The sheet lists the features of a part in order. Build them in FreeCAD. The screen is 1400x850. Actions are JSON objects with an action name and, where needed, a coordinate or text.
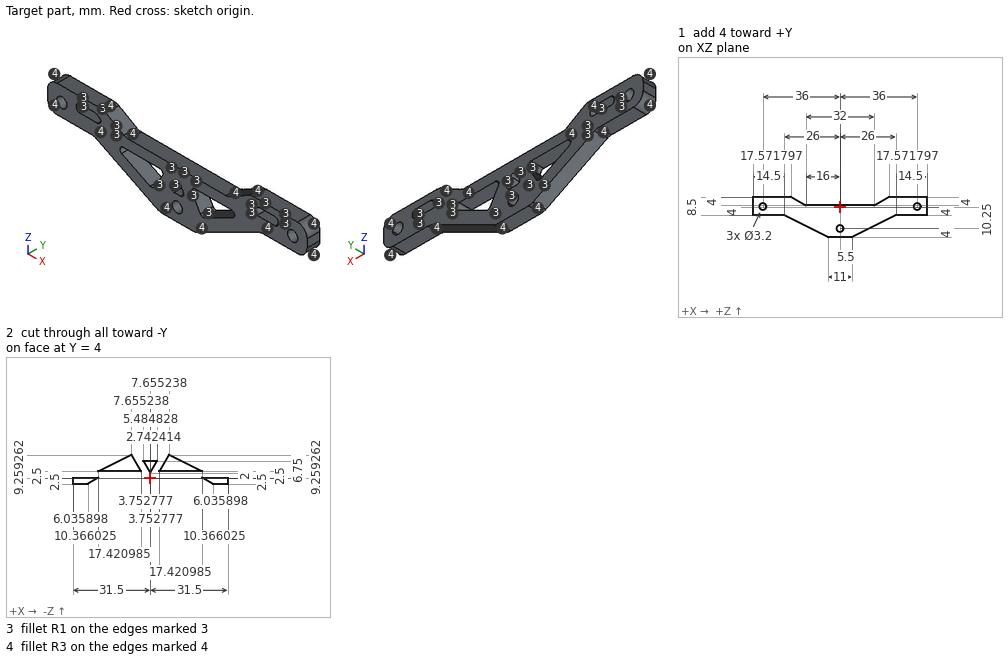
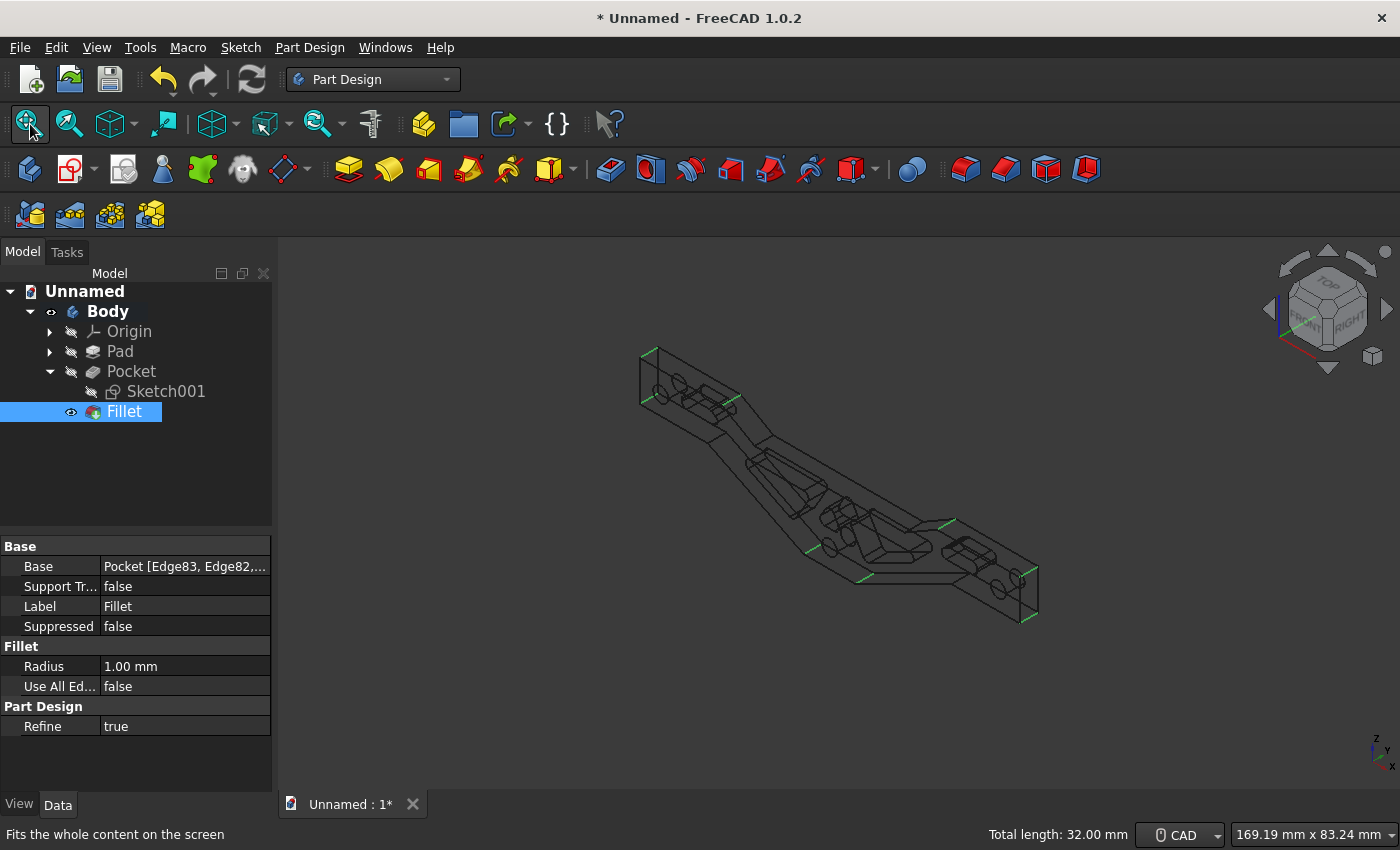
{"action": "left_click", "coordinate": [918, 524], "text": "ctrl"}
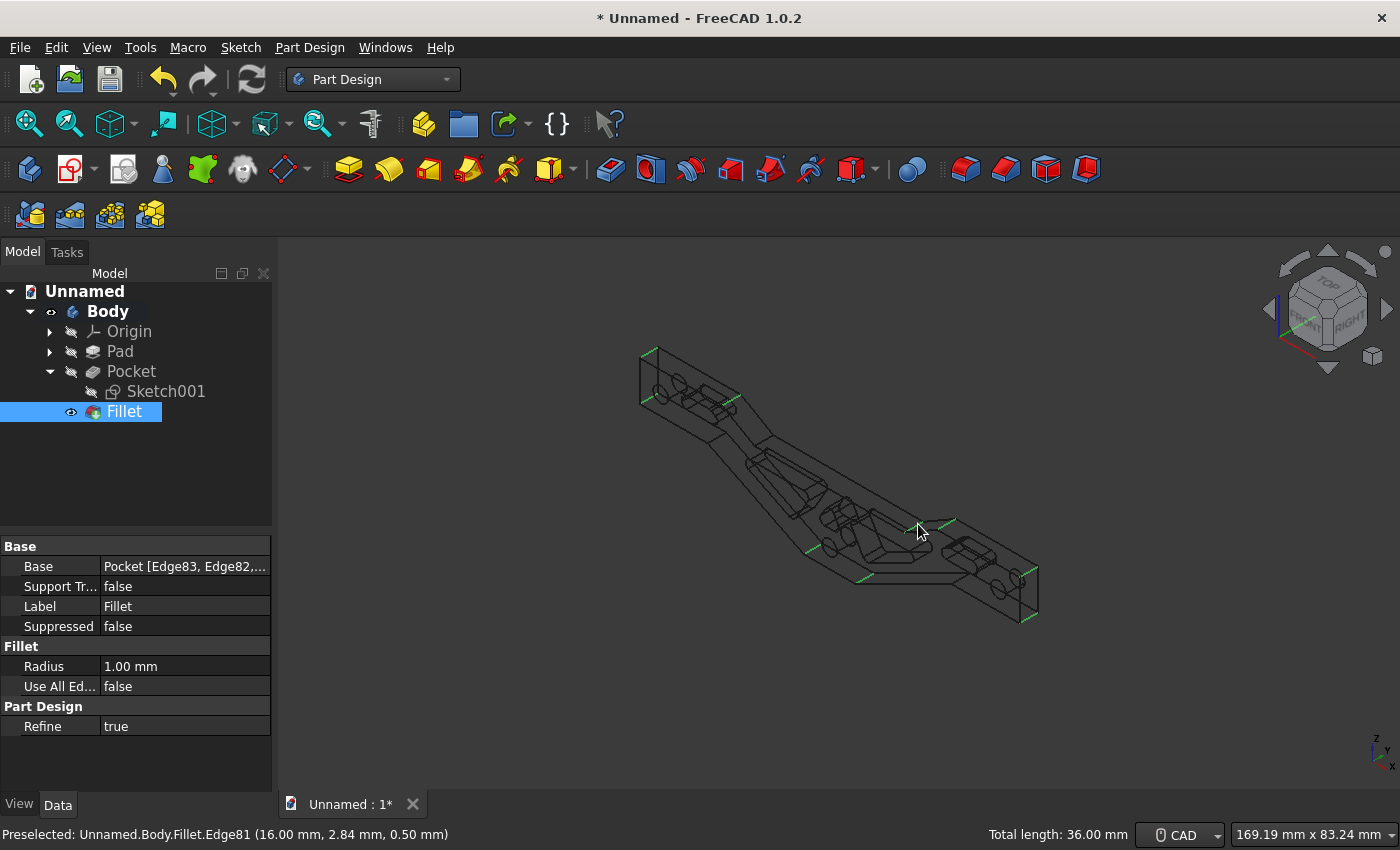
{"action": "left_click", "coordinate": [764, 440], "text": "ctrl"}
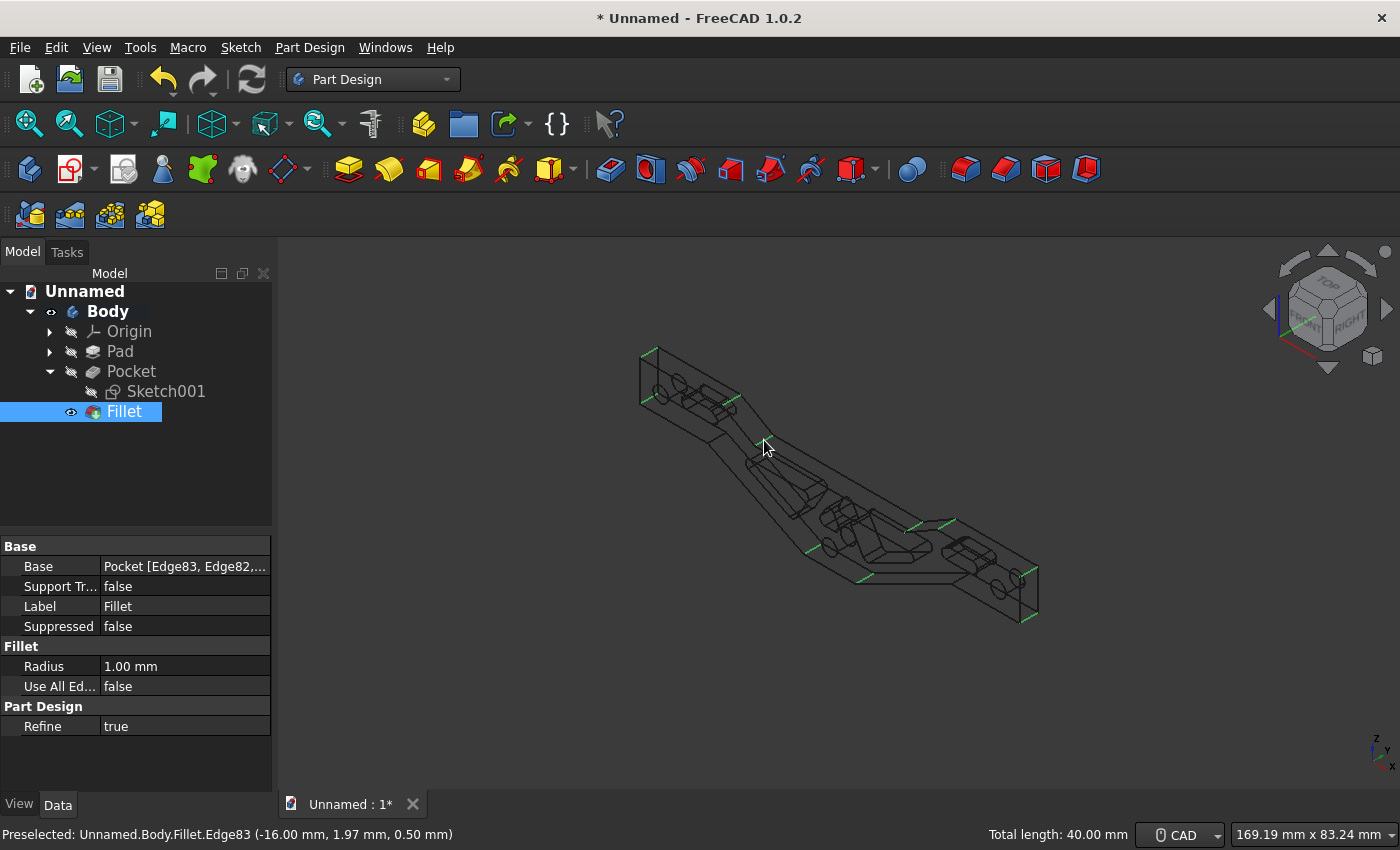
{"action": "left_click", "coordinate": [717, 437], "text": "ctrl"}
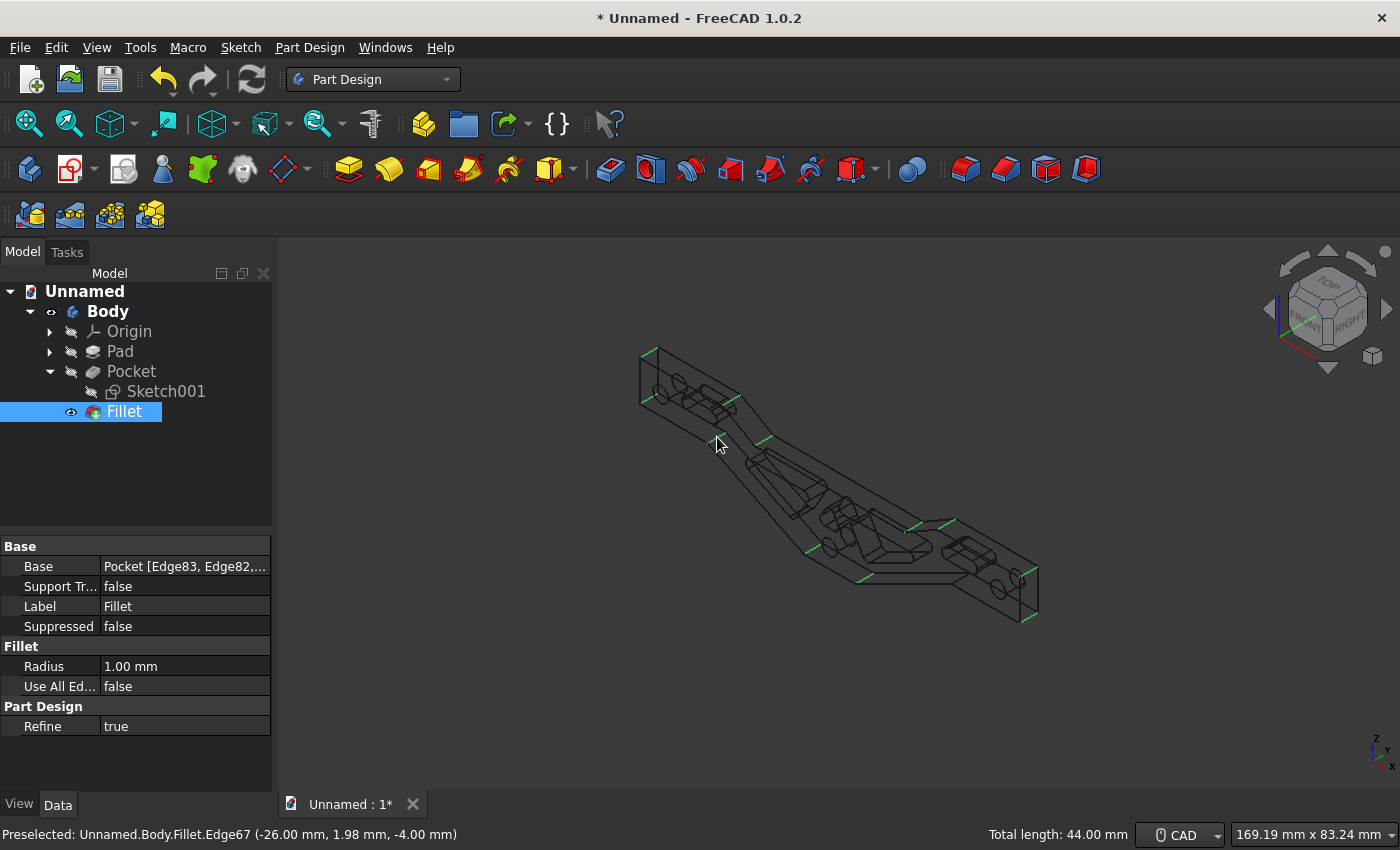
{"action": "left_click", "coordinate": [961, 578], "text": "ctrl"}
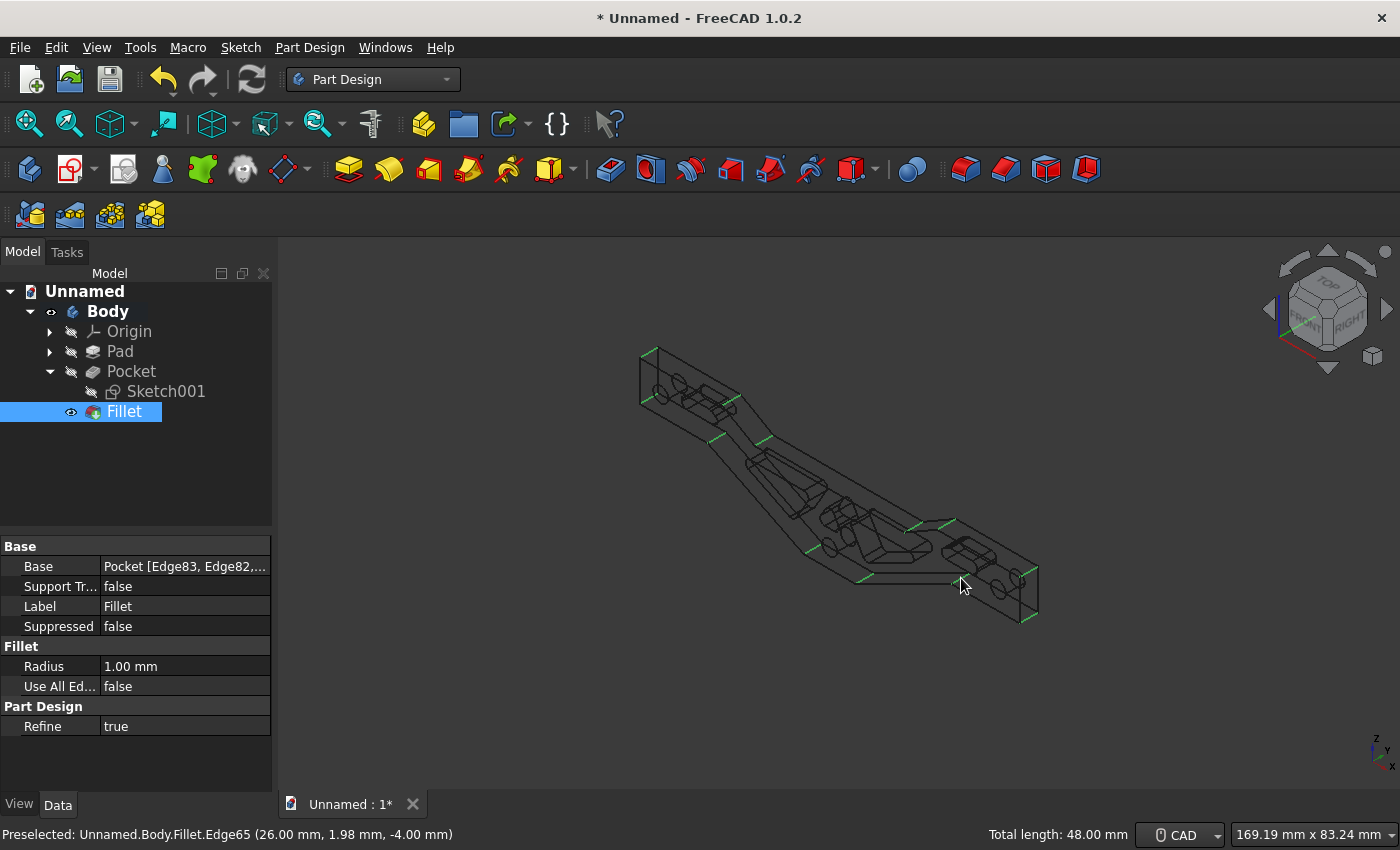
{"action": "key", "text": "v 1"}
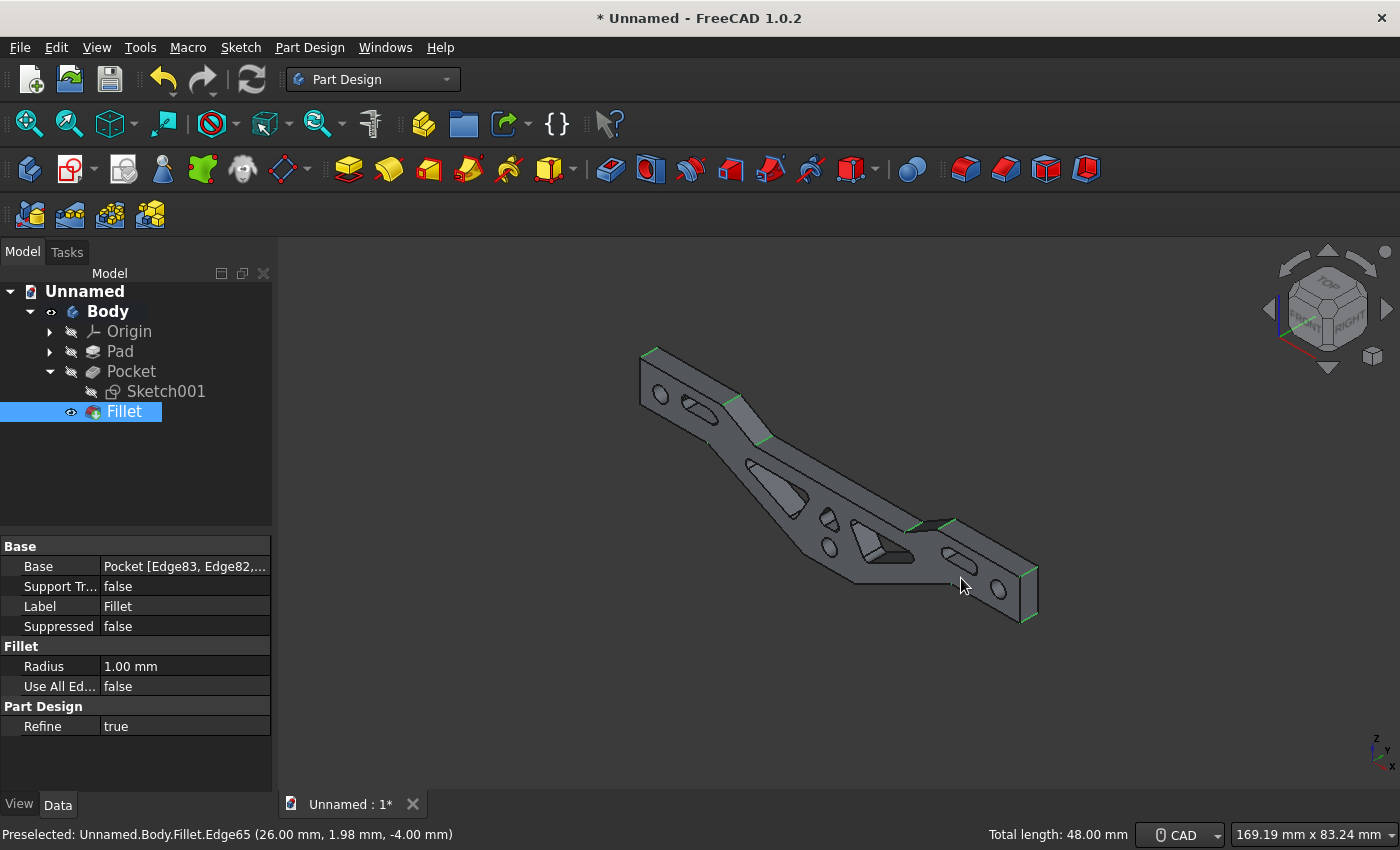
{"action": "left_click", "coordinate": [966, 170]}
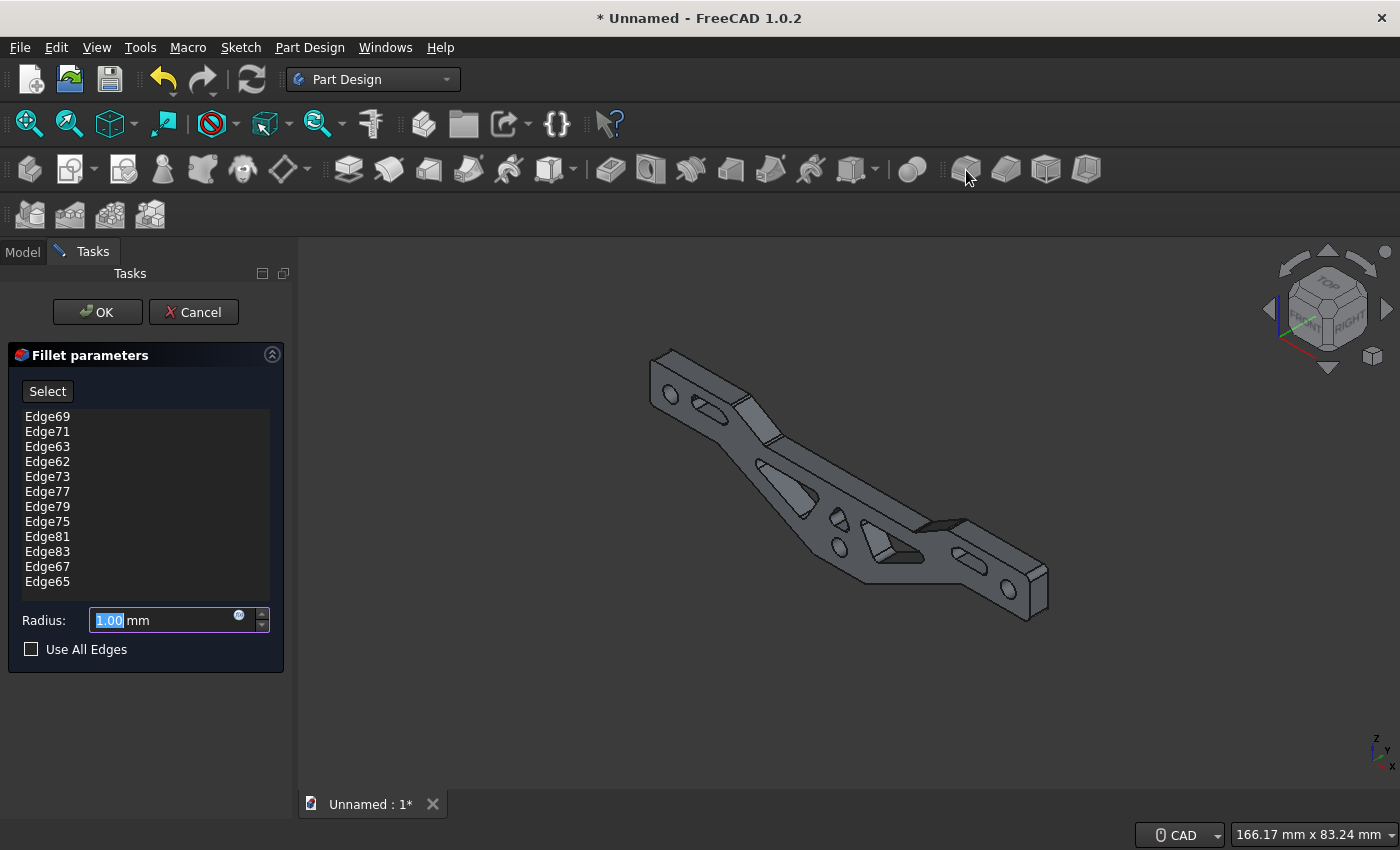
{"action": "type", "text": "3"}
{"action": "key", "text": "Tab"}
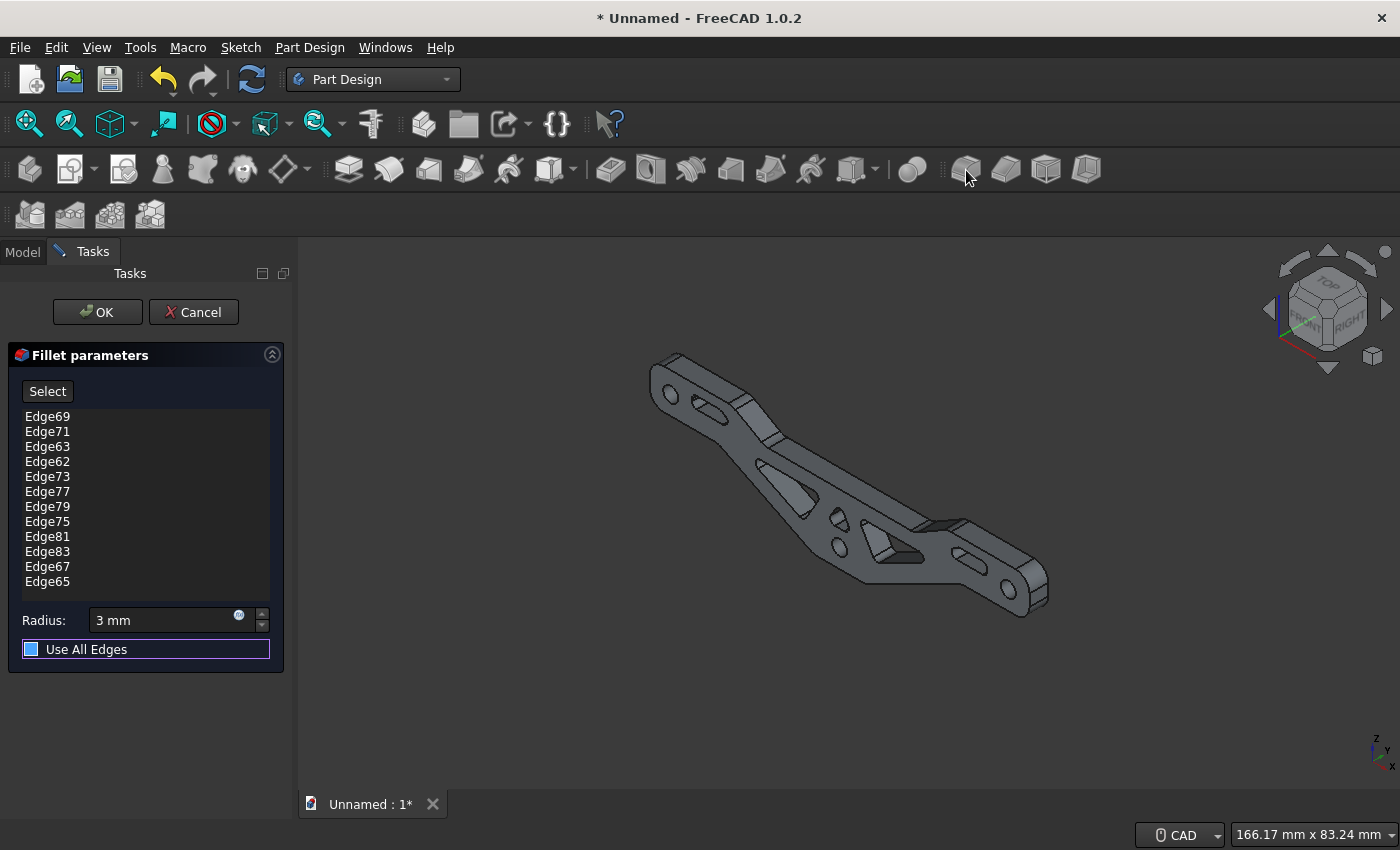
{"action": "left_click", "coordinate": [98, 312]}